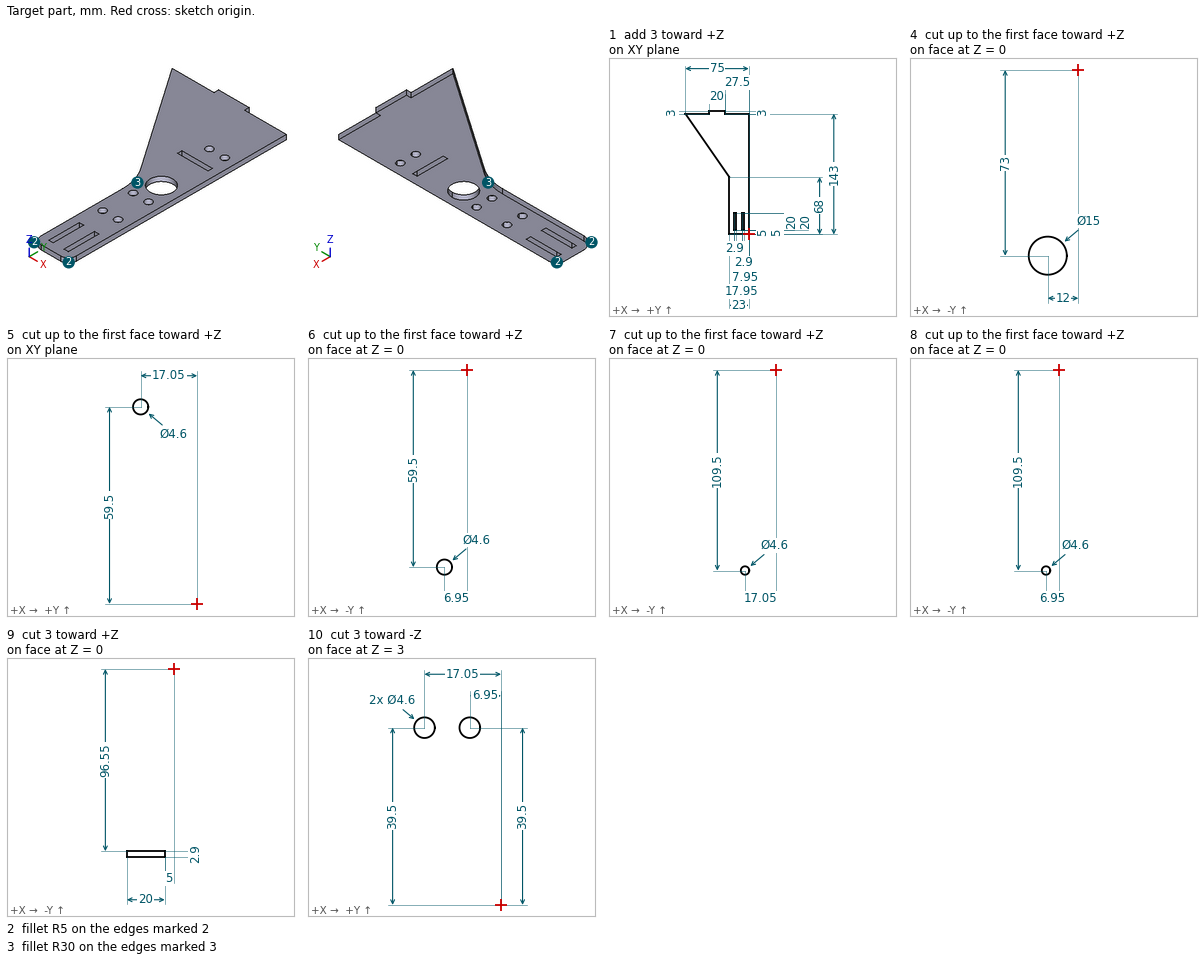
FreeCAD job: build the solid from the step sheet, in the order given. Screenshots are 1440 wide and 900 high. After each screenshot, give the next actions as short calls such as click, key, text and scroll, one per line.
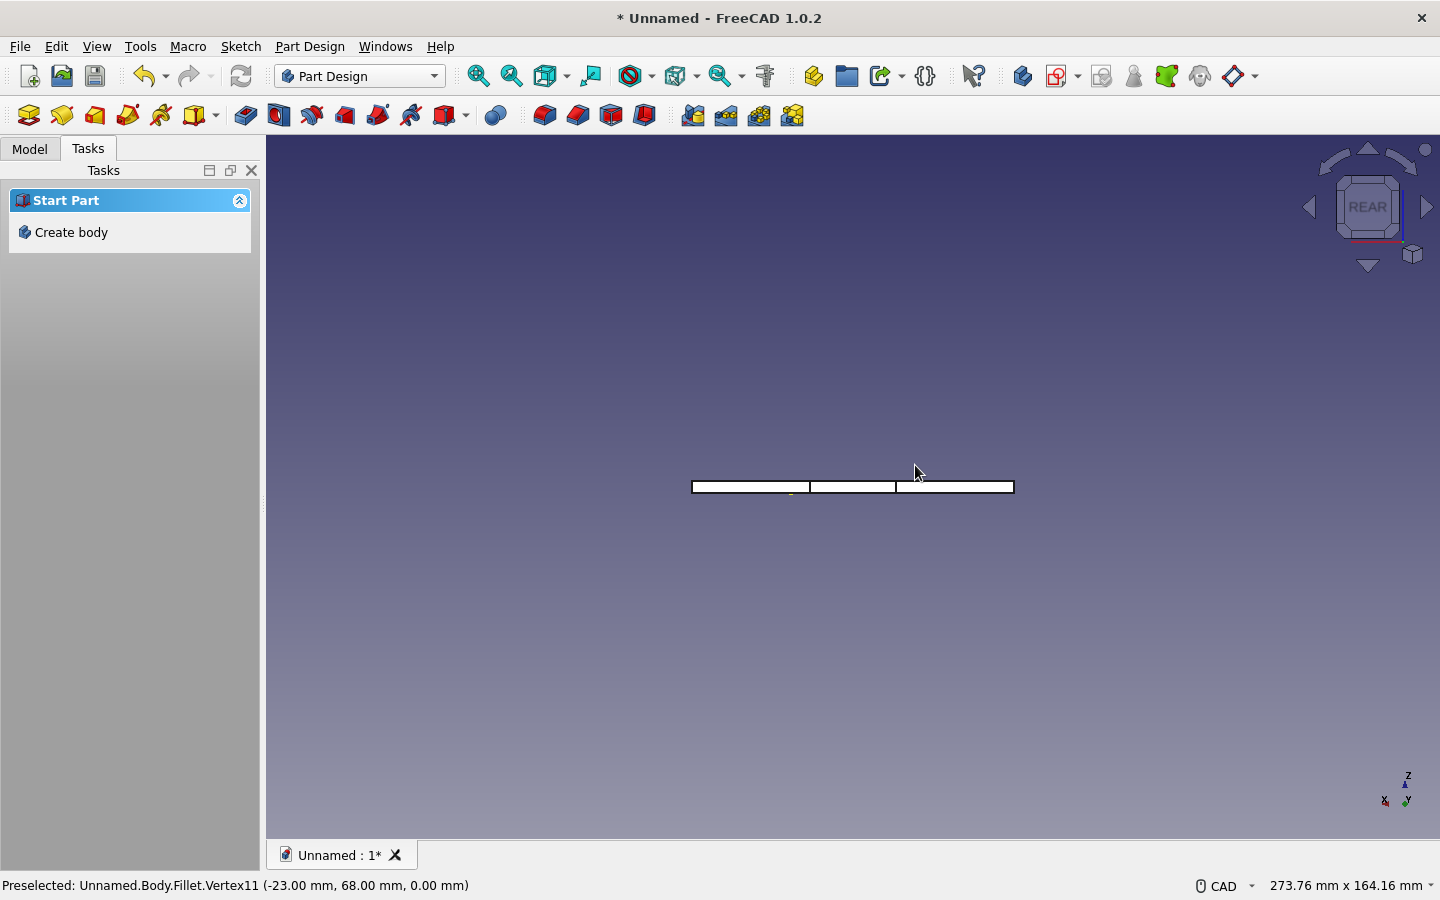
scroll(791, 486, up, 6)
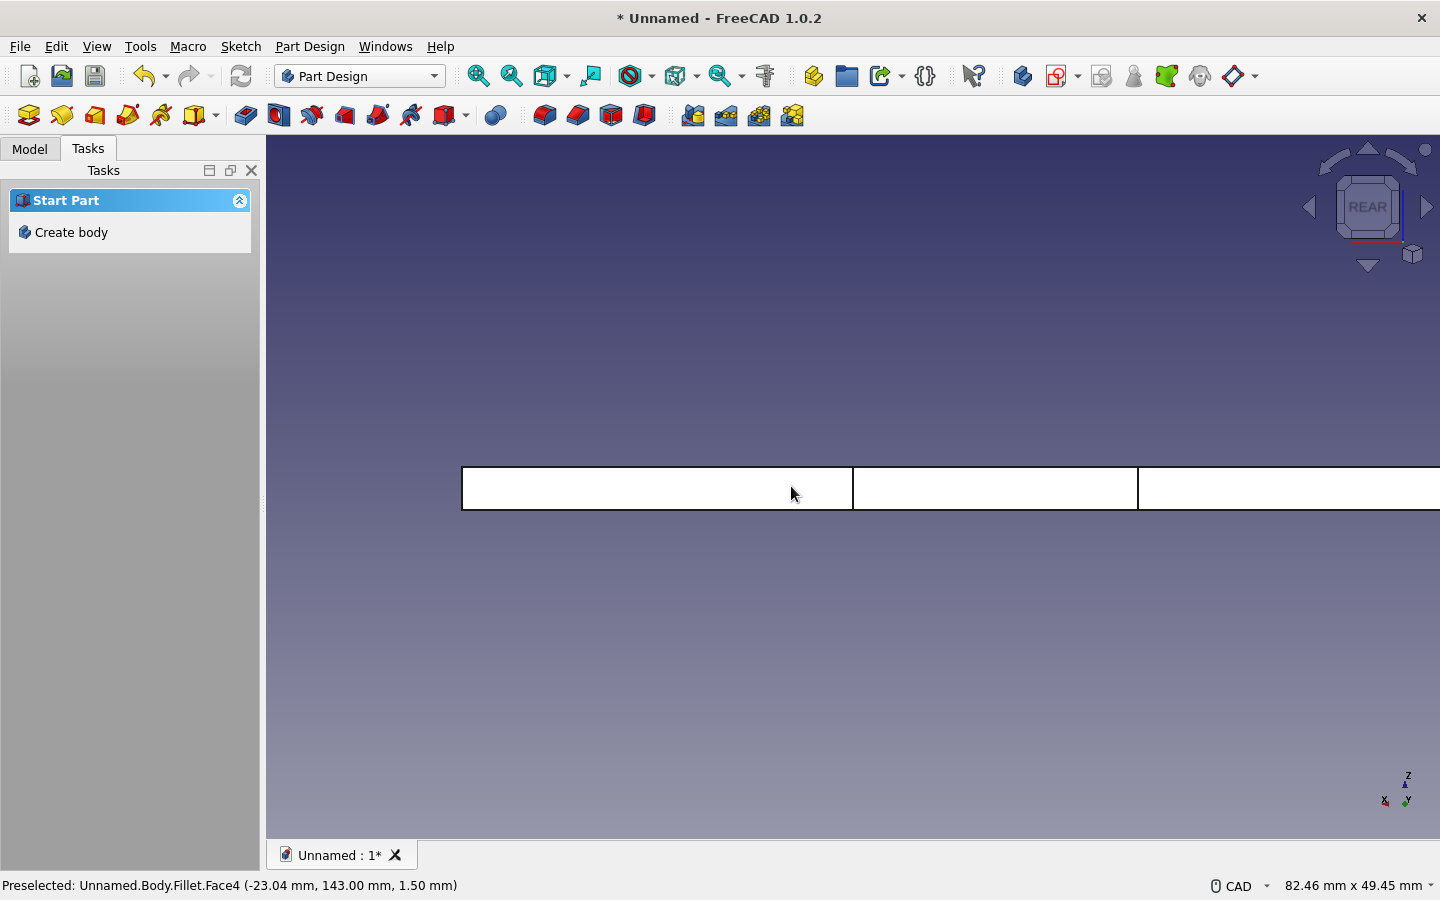
click(479, 76)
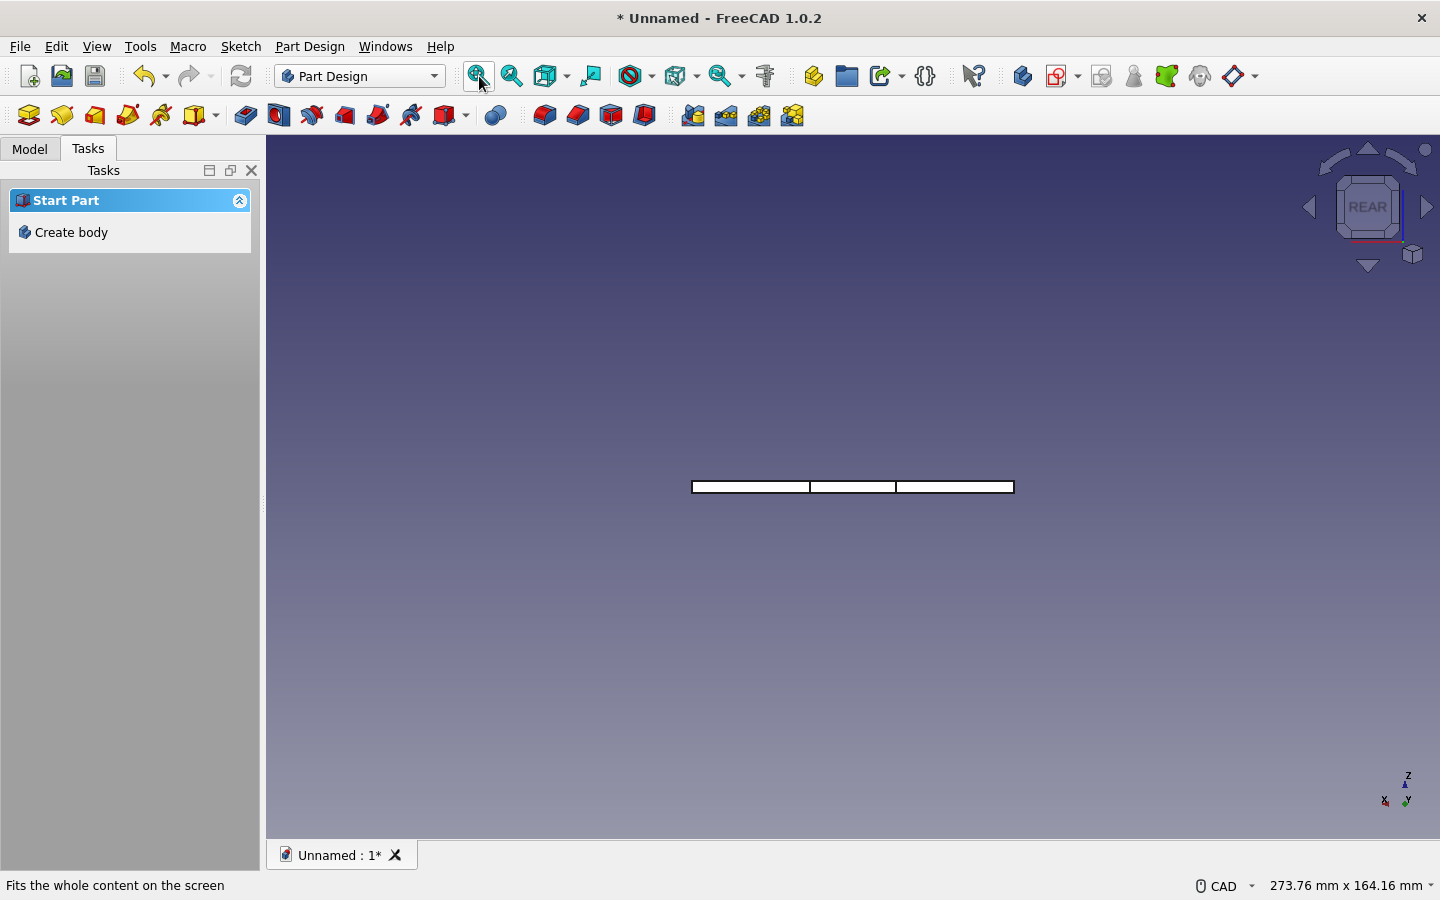
key(6)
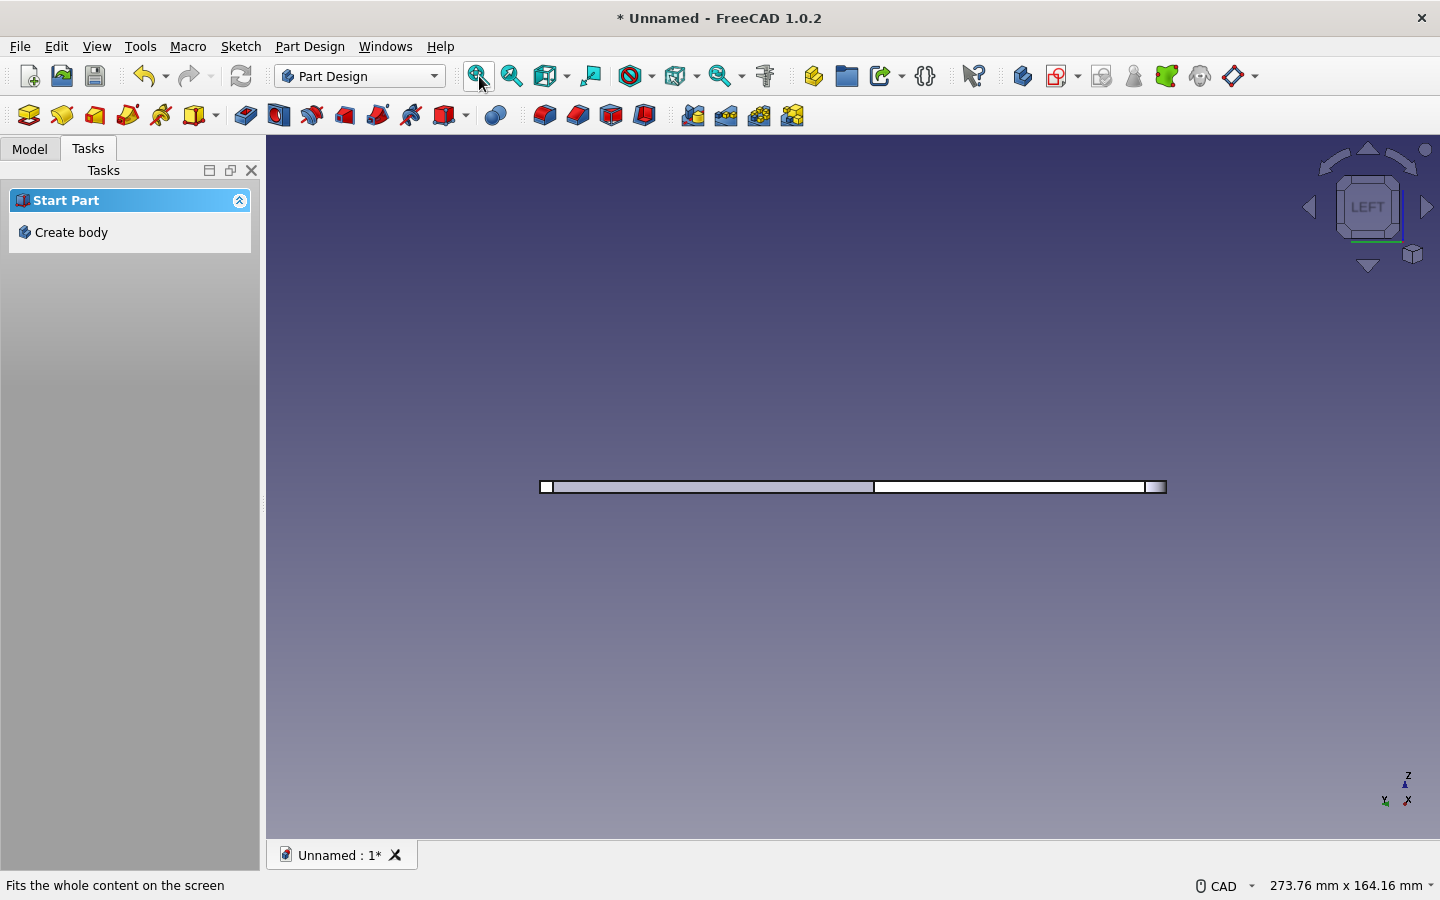
scroll(874, 486, up, 6)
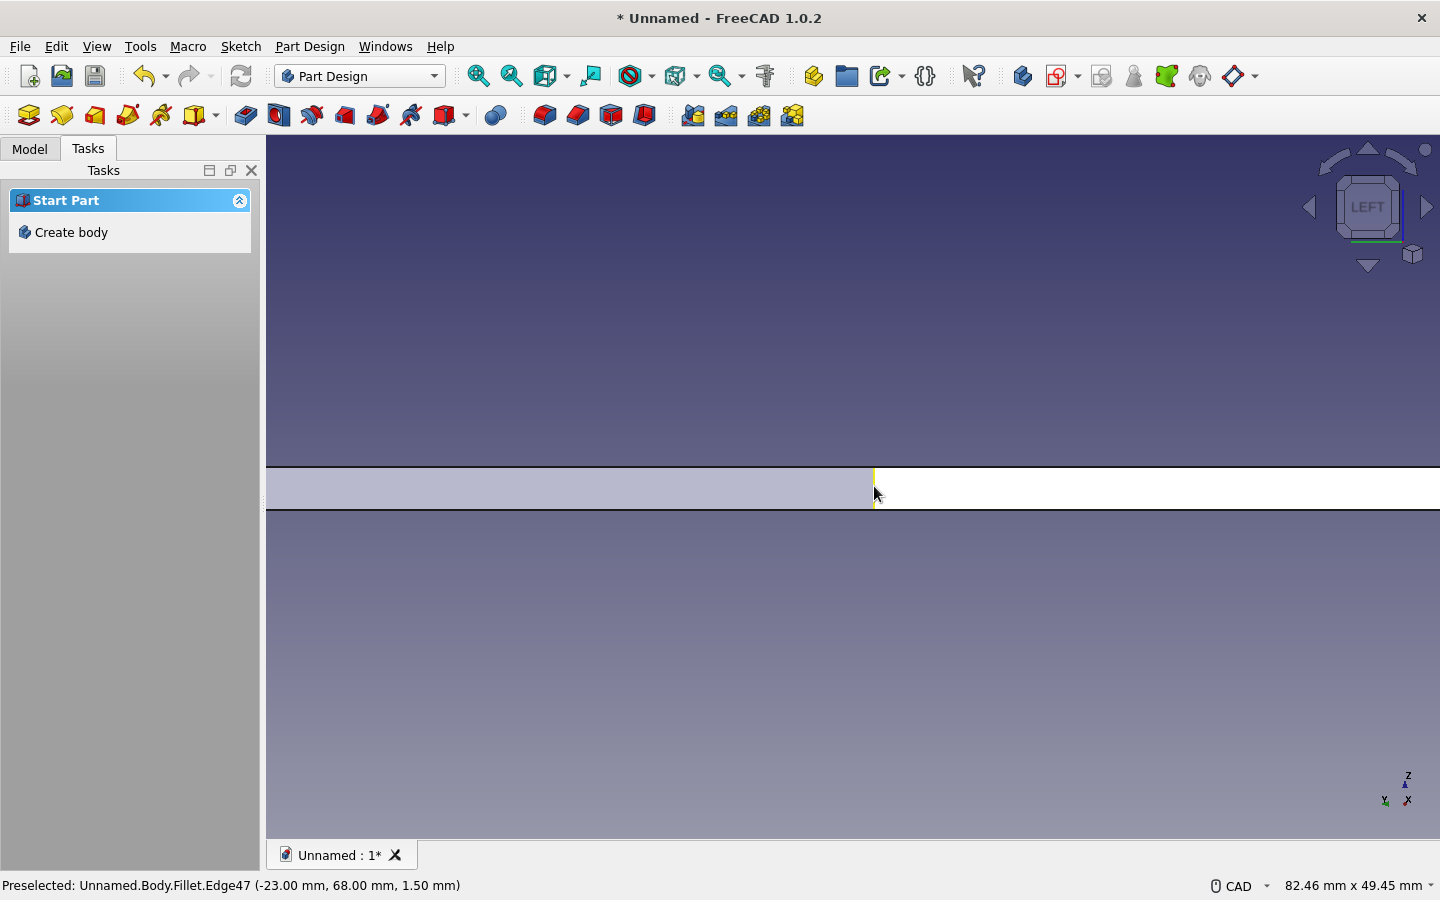
key(v)
key(f)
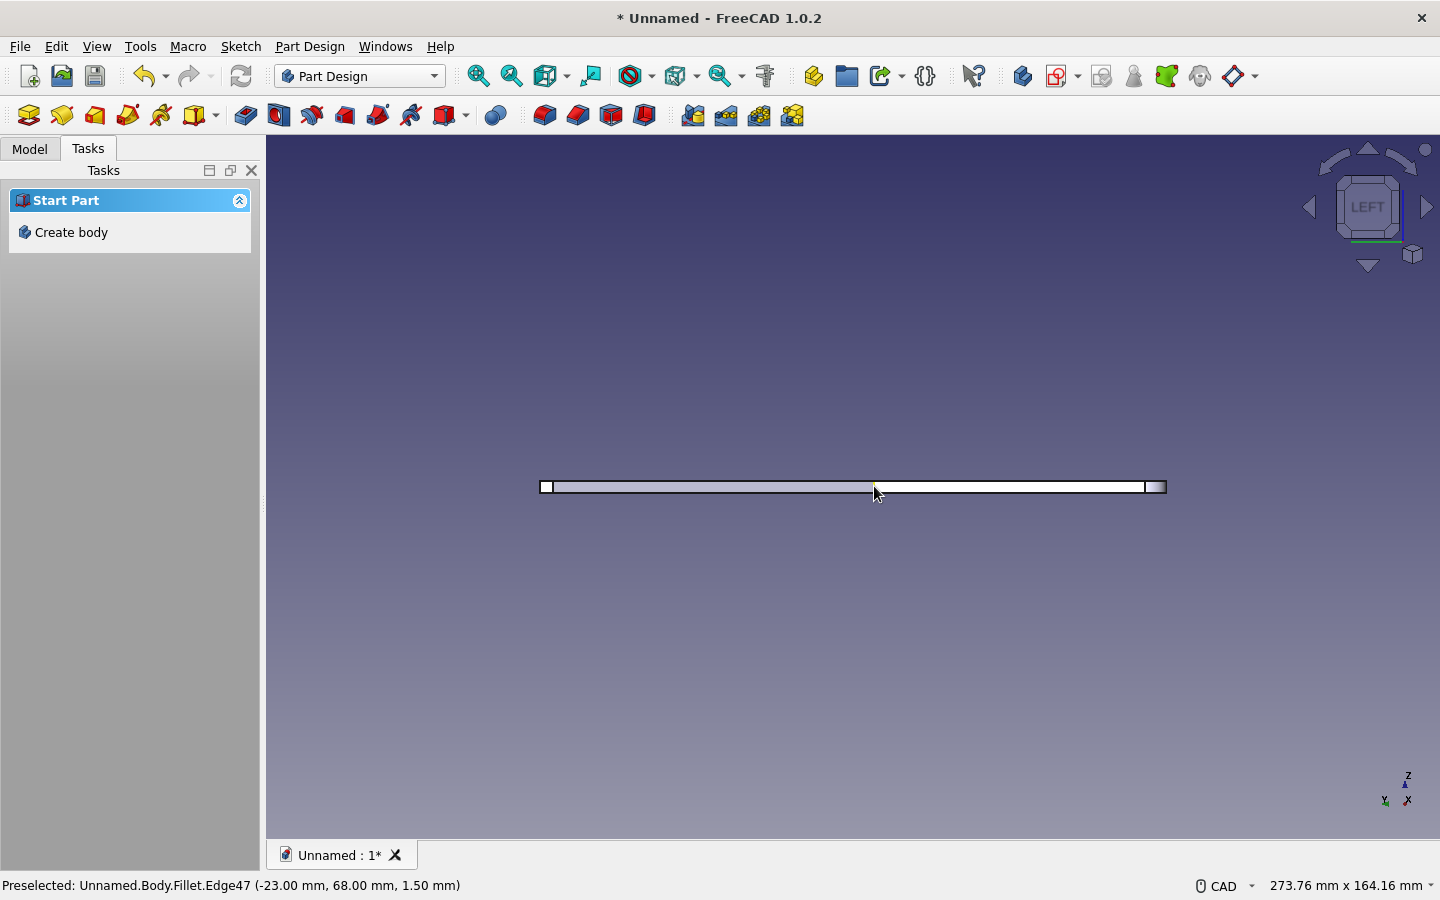
key(v)
key(3)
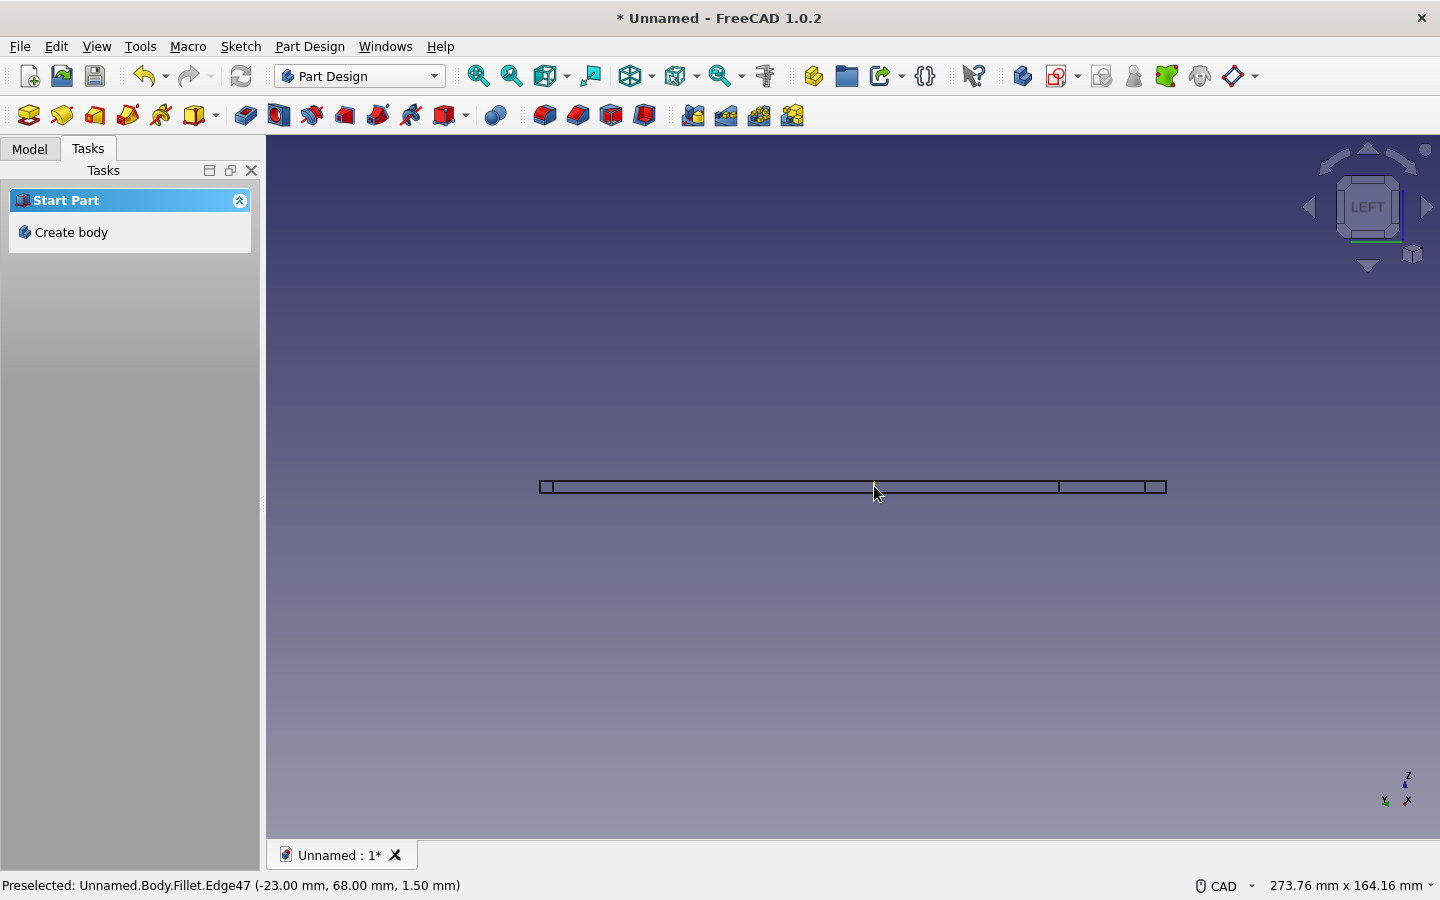
key(0)